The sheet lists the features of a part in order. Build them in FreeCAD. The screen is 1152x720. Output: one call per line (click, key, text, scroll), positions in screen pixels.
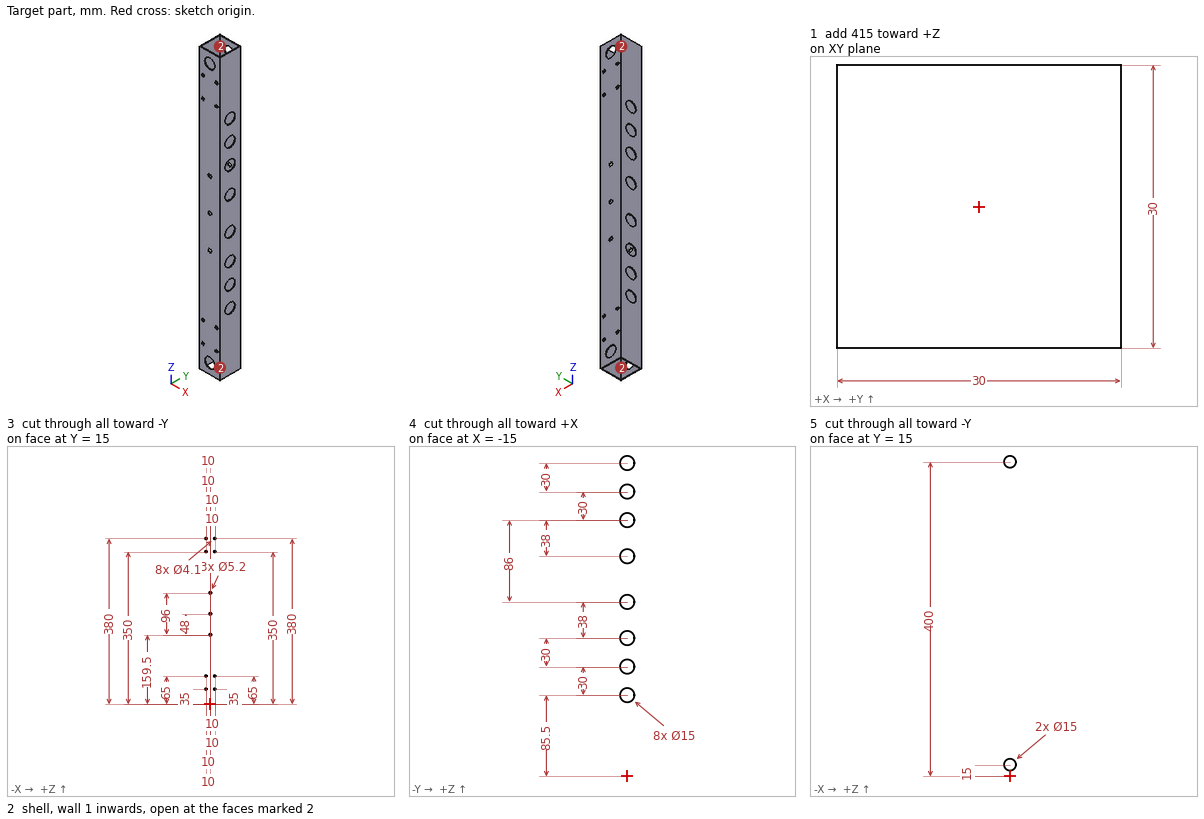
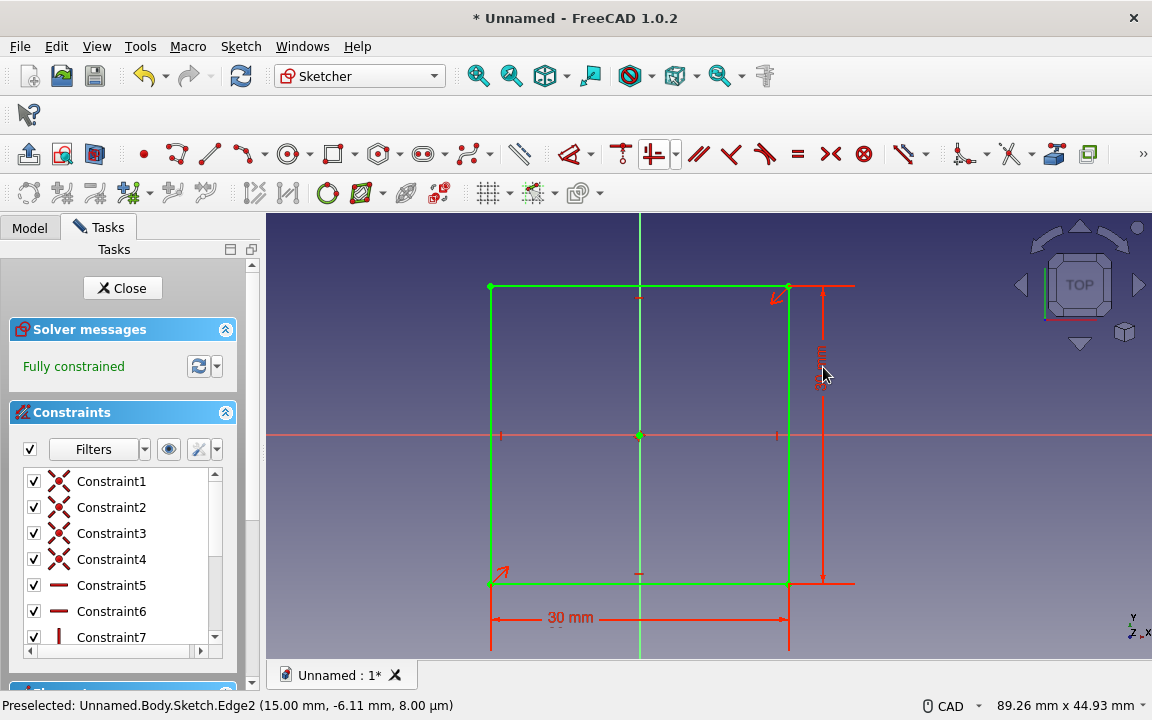
click(123, 288)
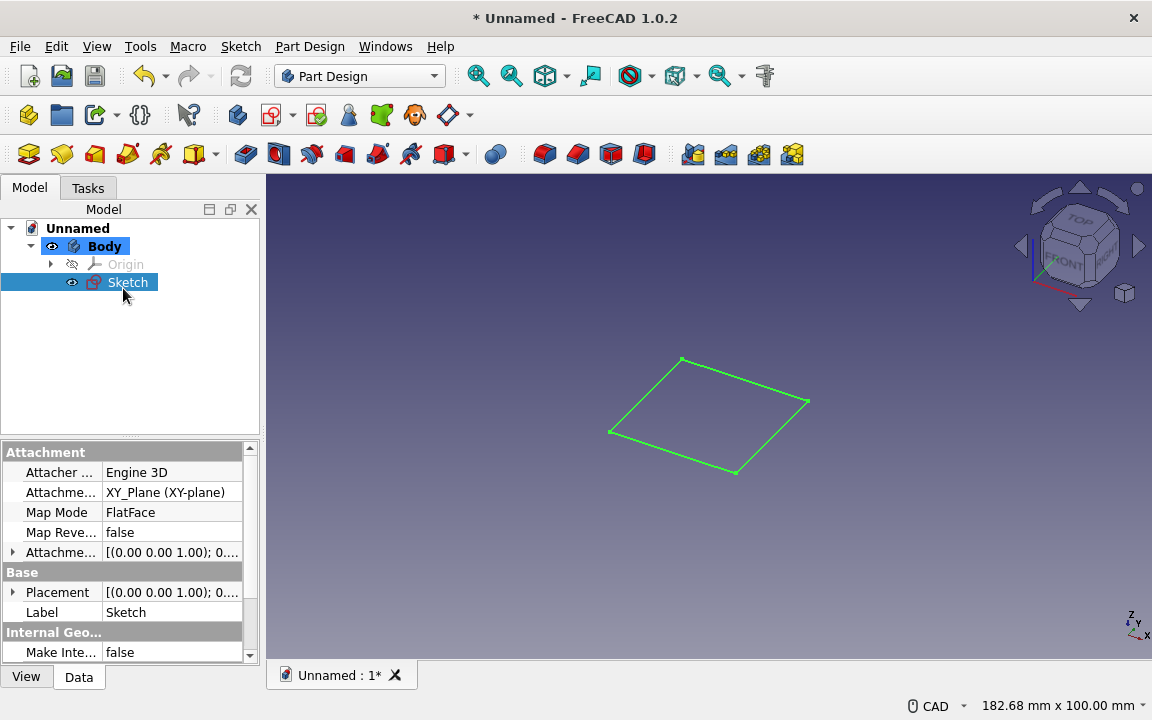
click(29, 154)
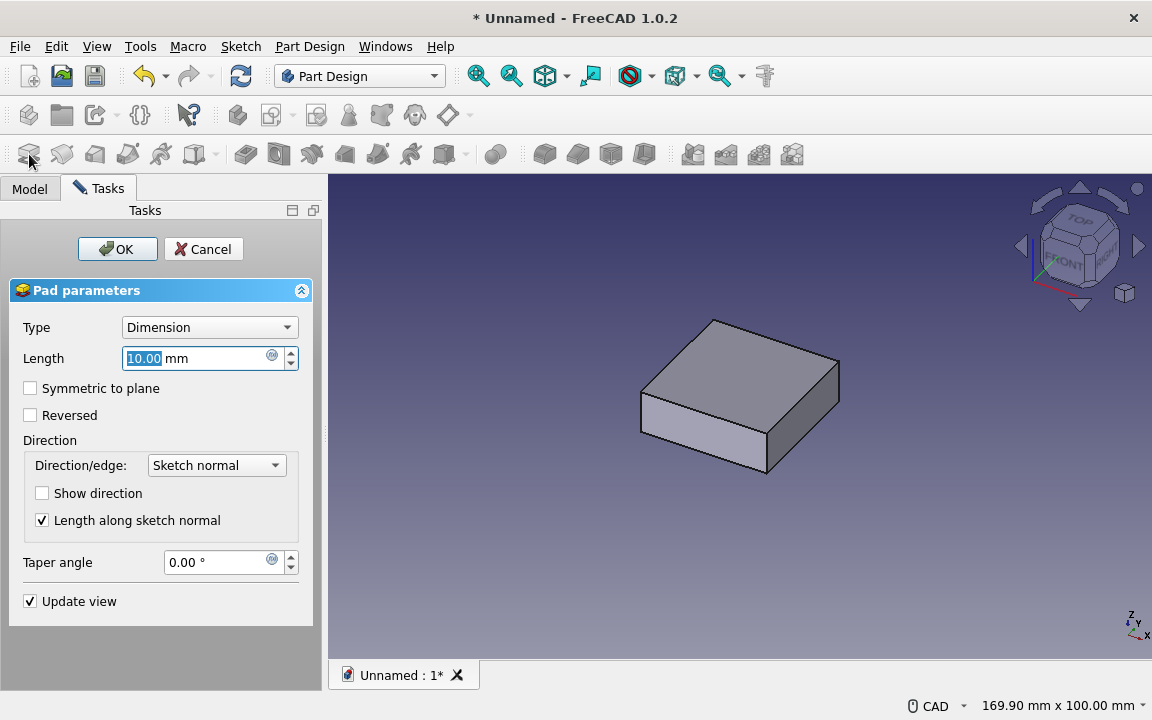
text(415)
key(Tab)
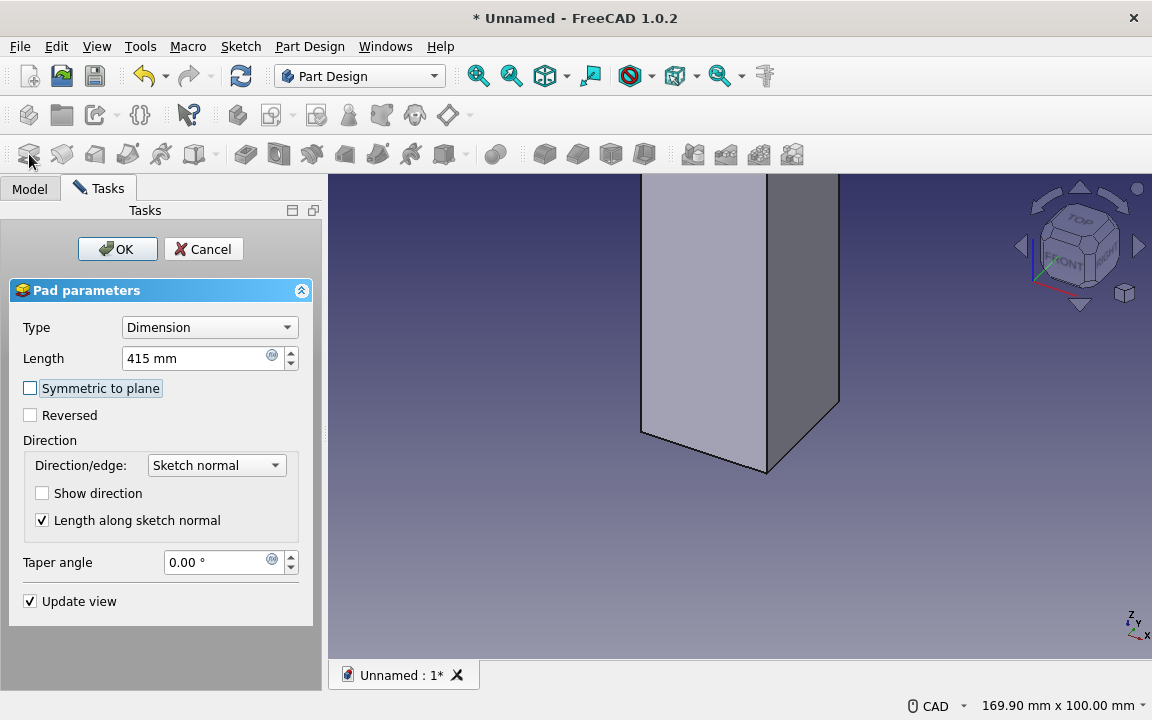
click(118, 249)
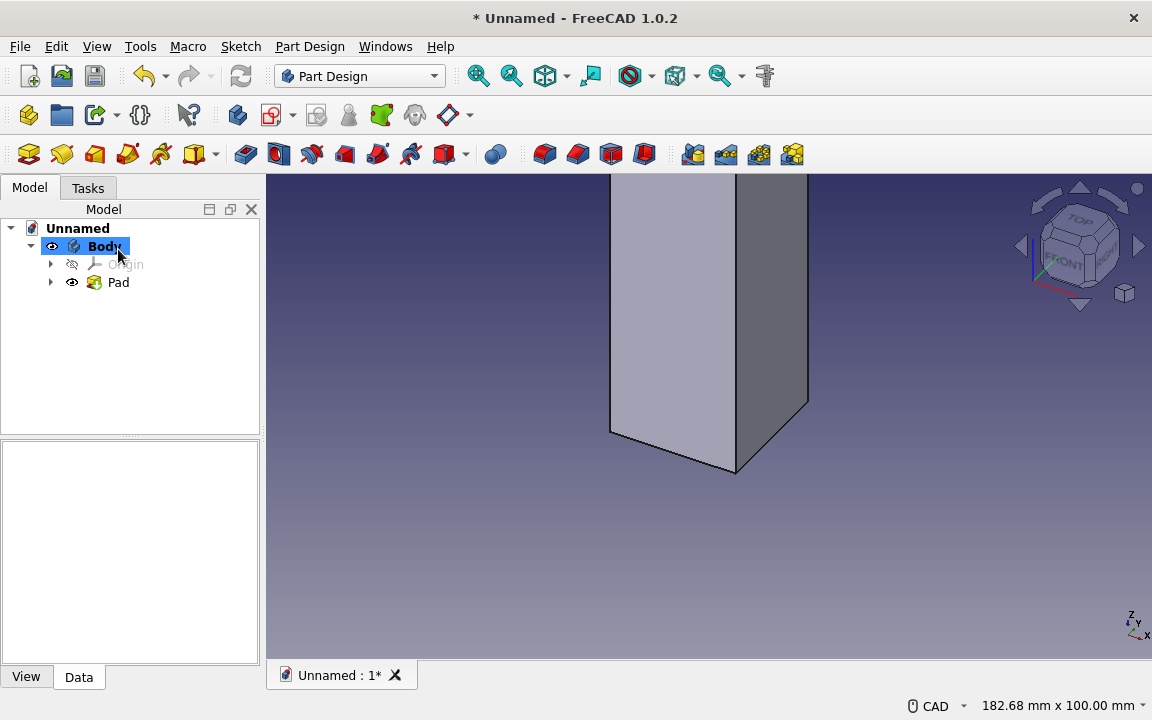
key(v)
key(f)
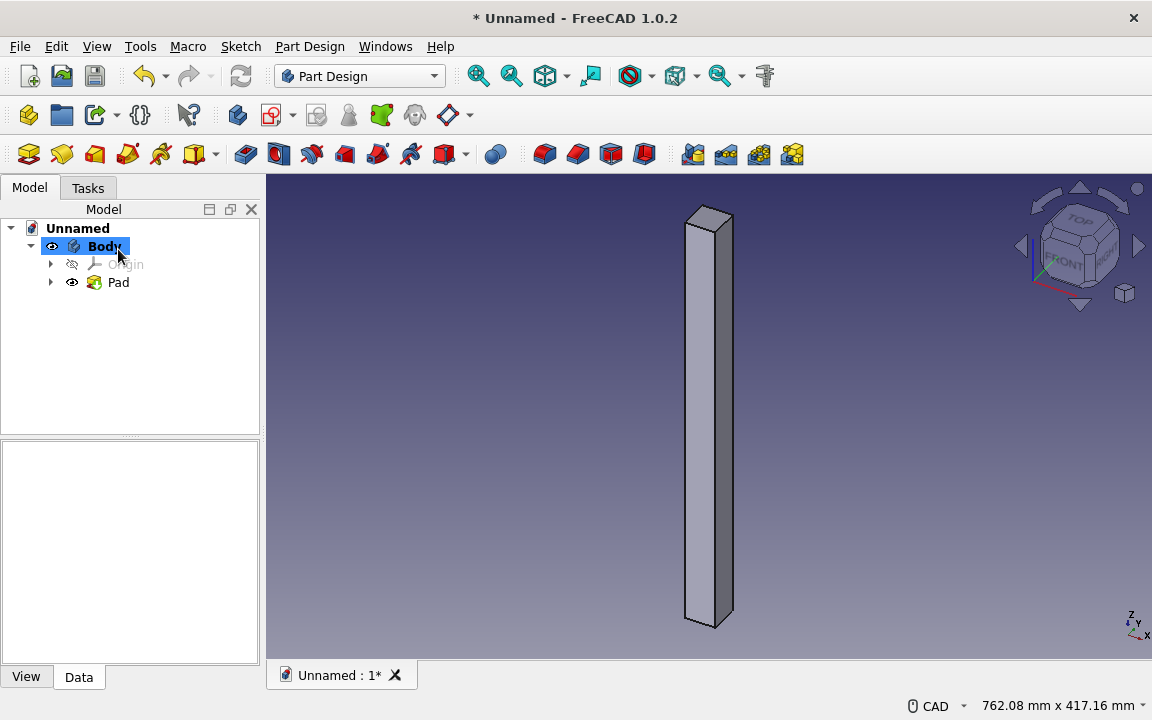
click(709, 218)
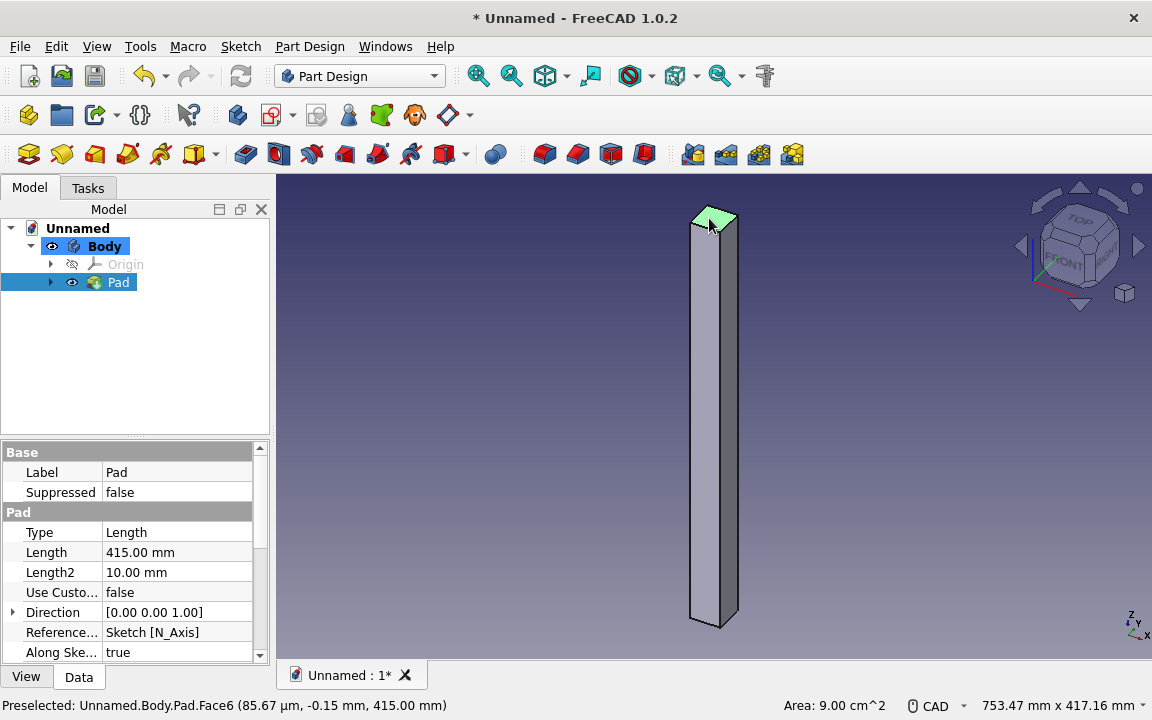
key(0)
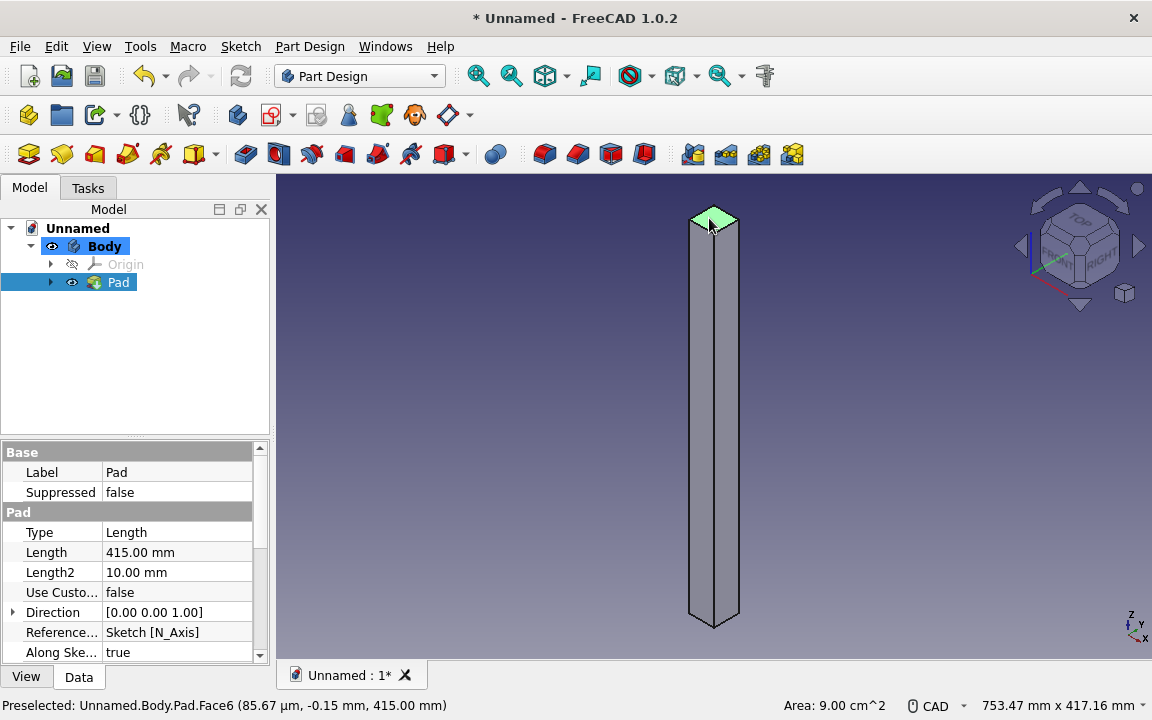
key(2)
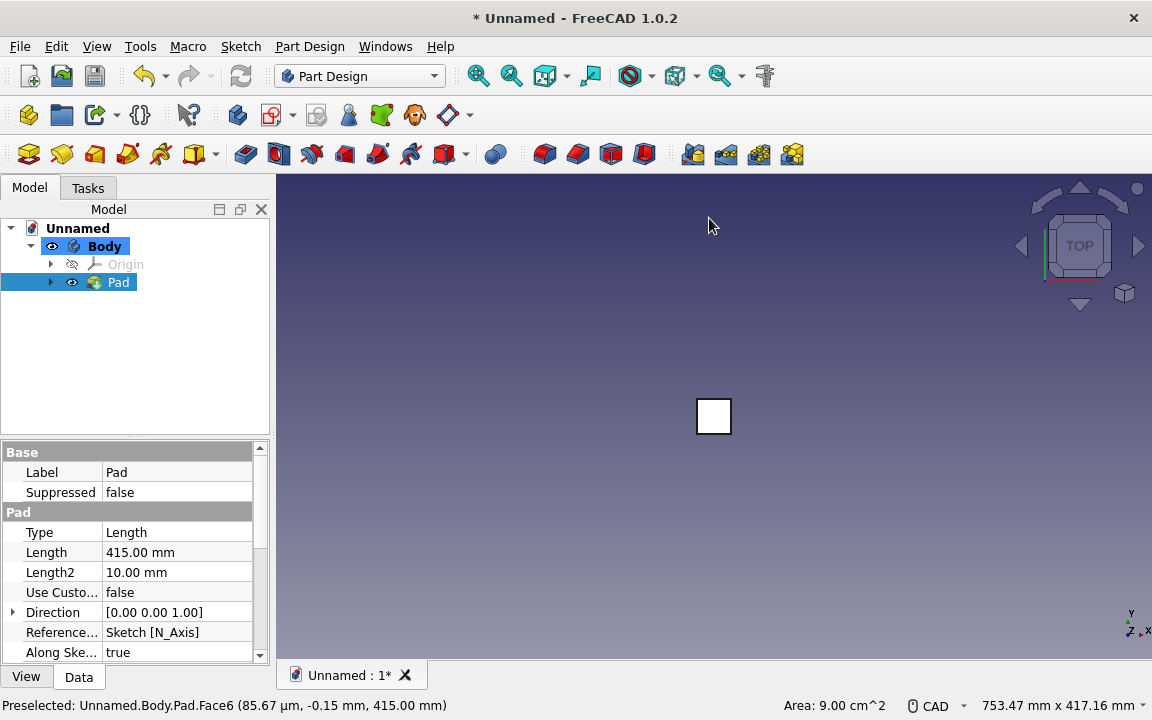
click(479, 76)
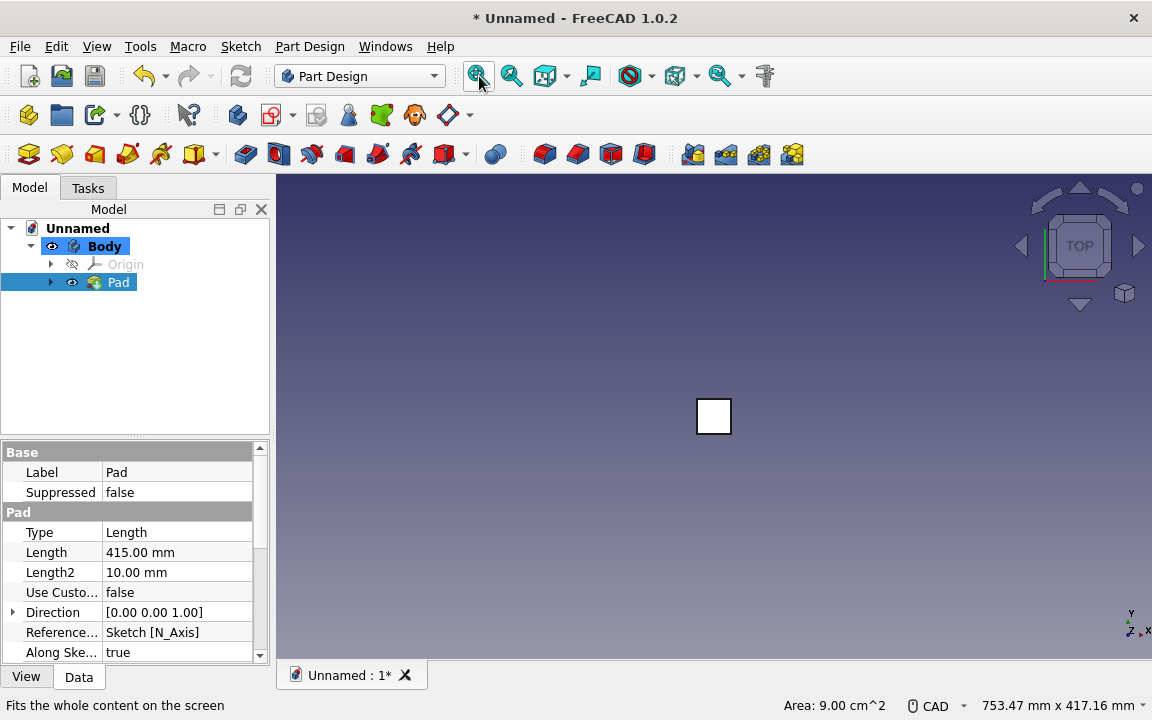
key(1)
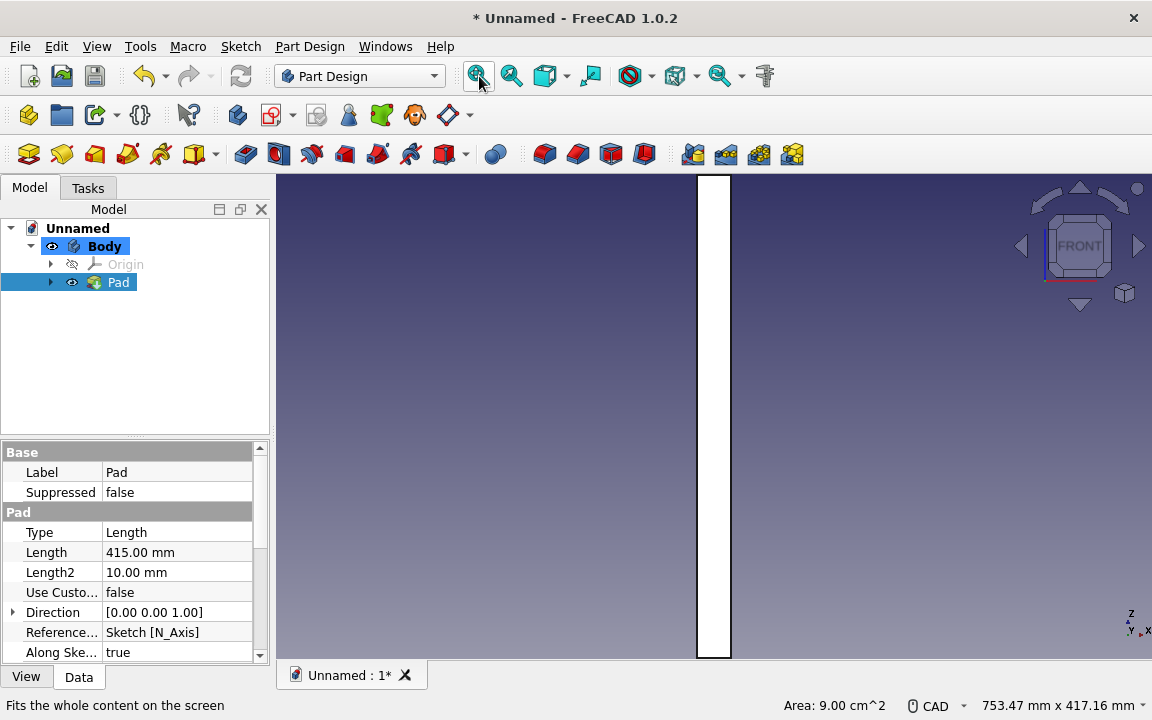
key(3)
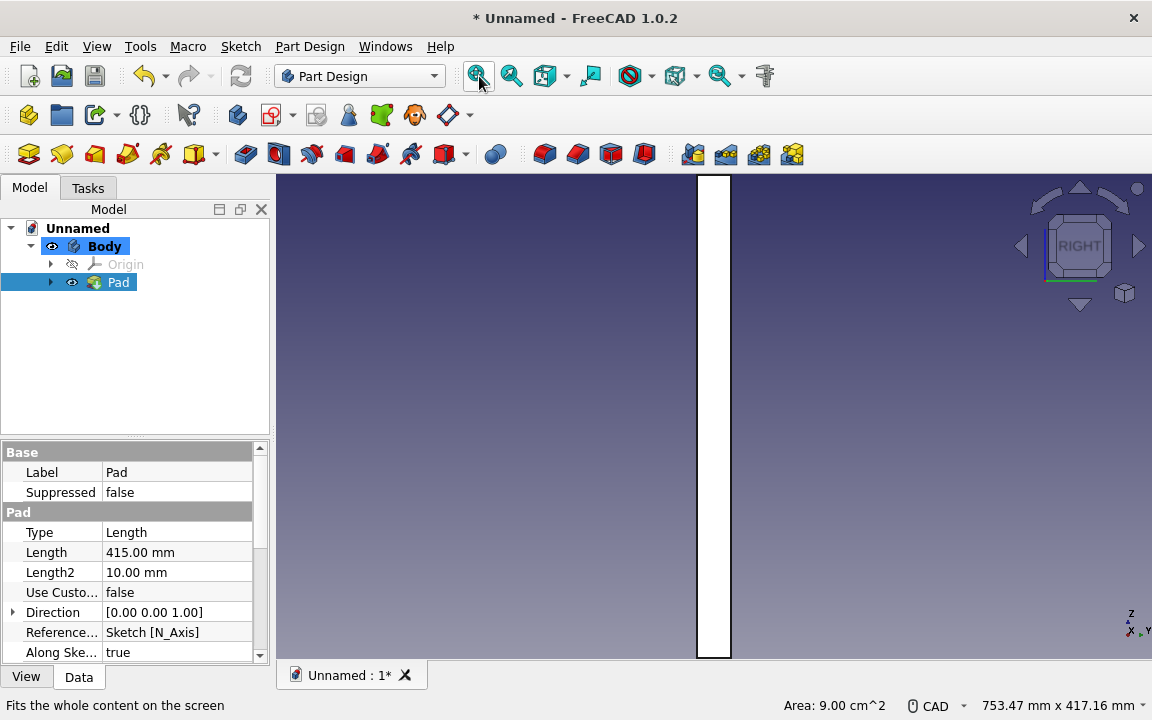
key(5)